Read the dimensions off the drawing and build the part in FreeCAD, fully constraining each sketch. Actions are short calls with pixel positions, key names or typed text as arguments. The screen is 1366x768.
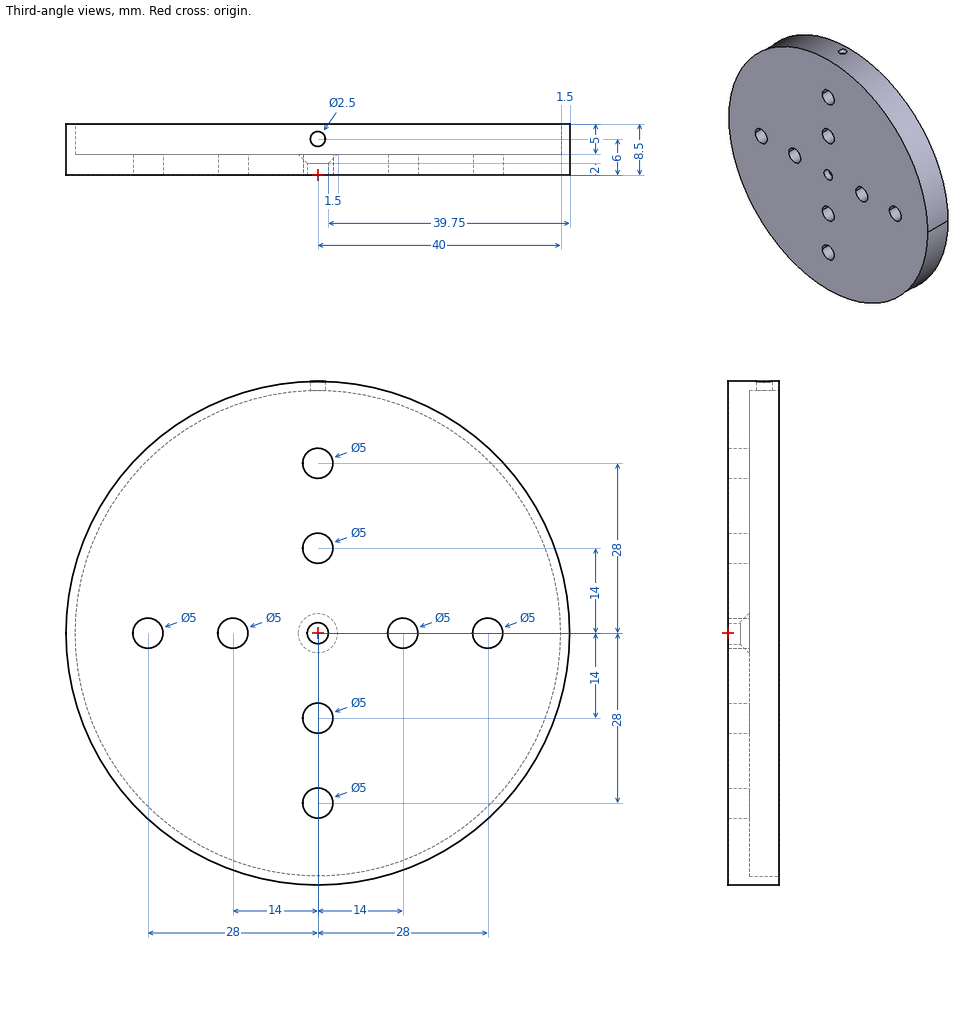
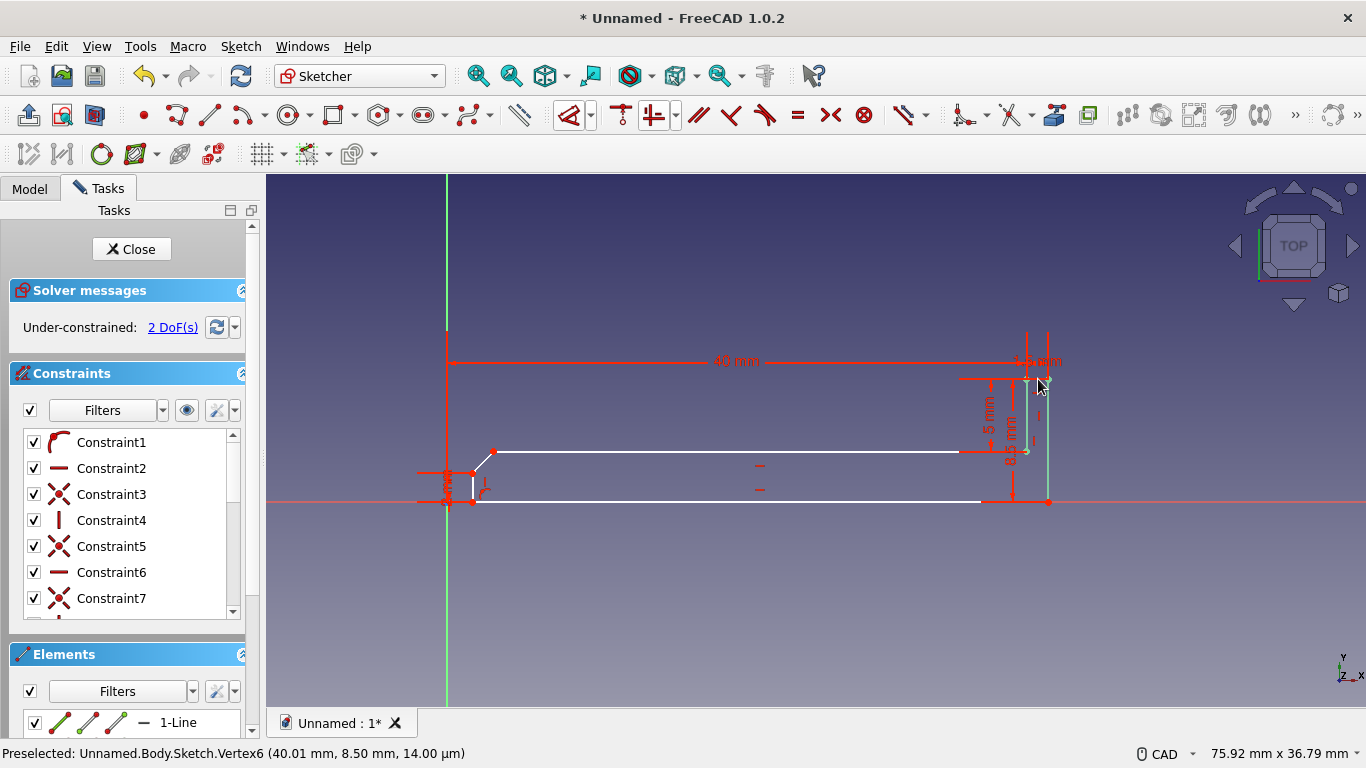
scroll(487, 458, up, 4)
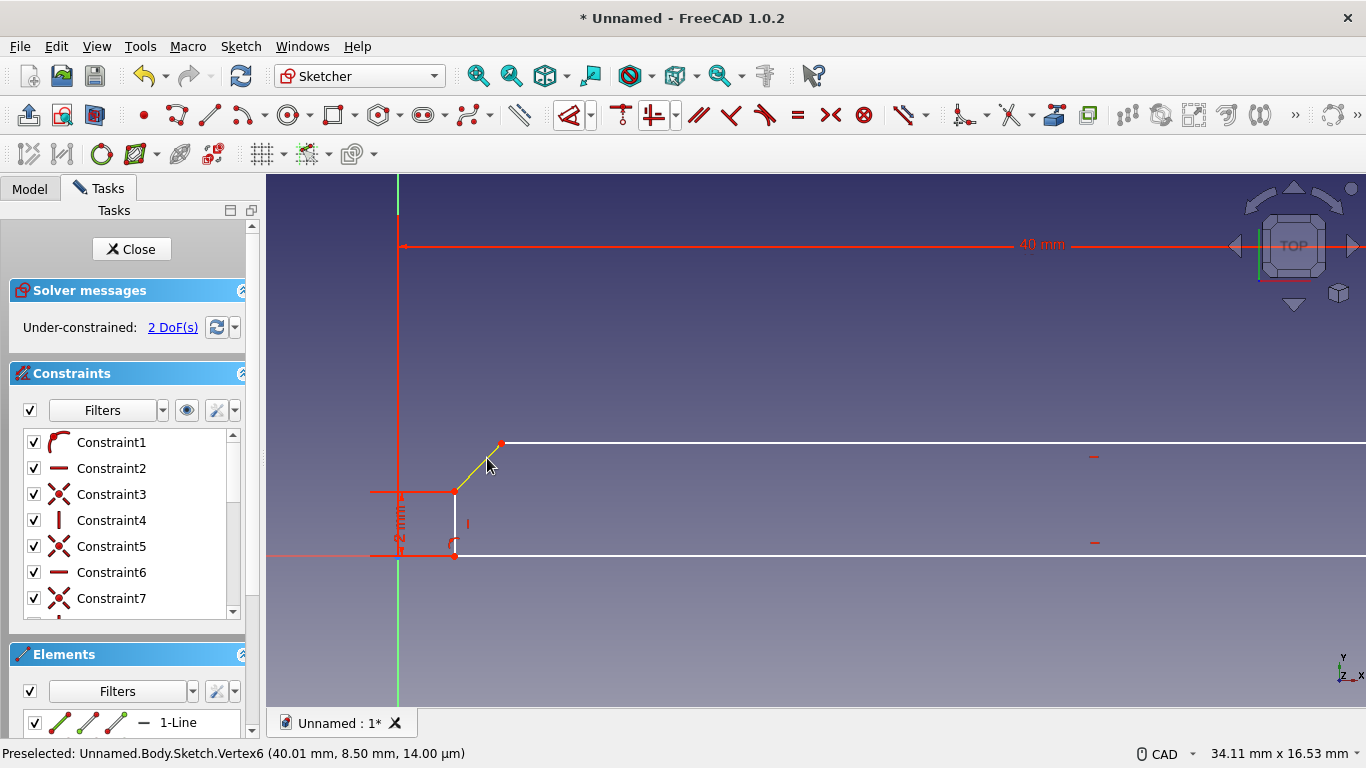
click(488, 458)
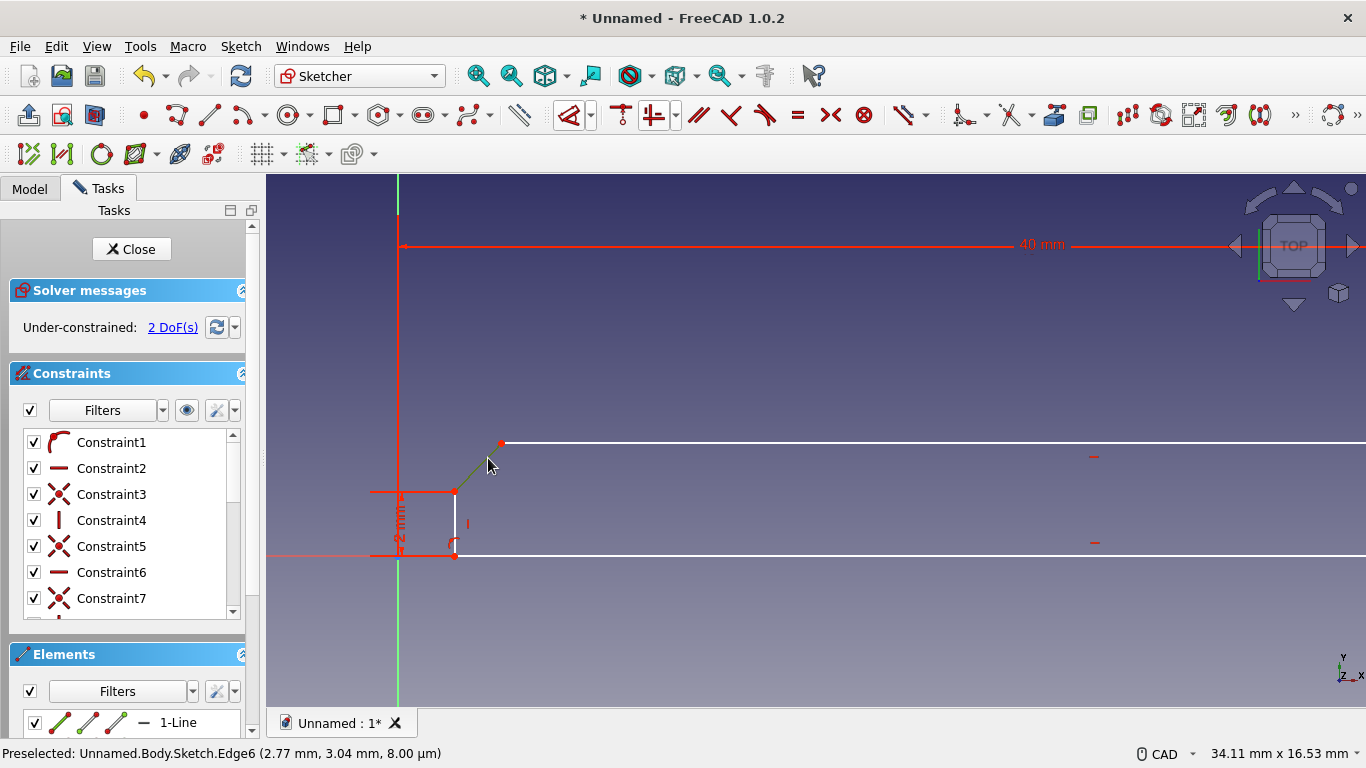
click(590, 116)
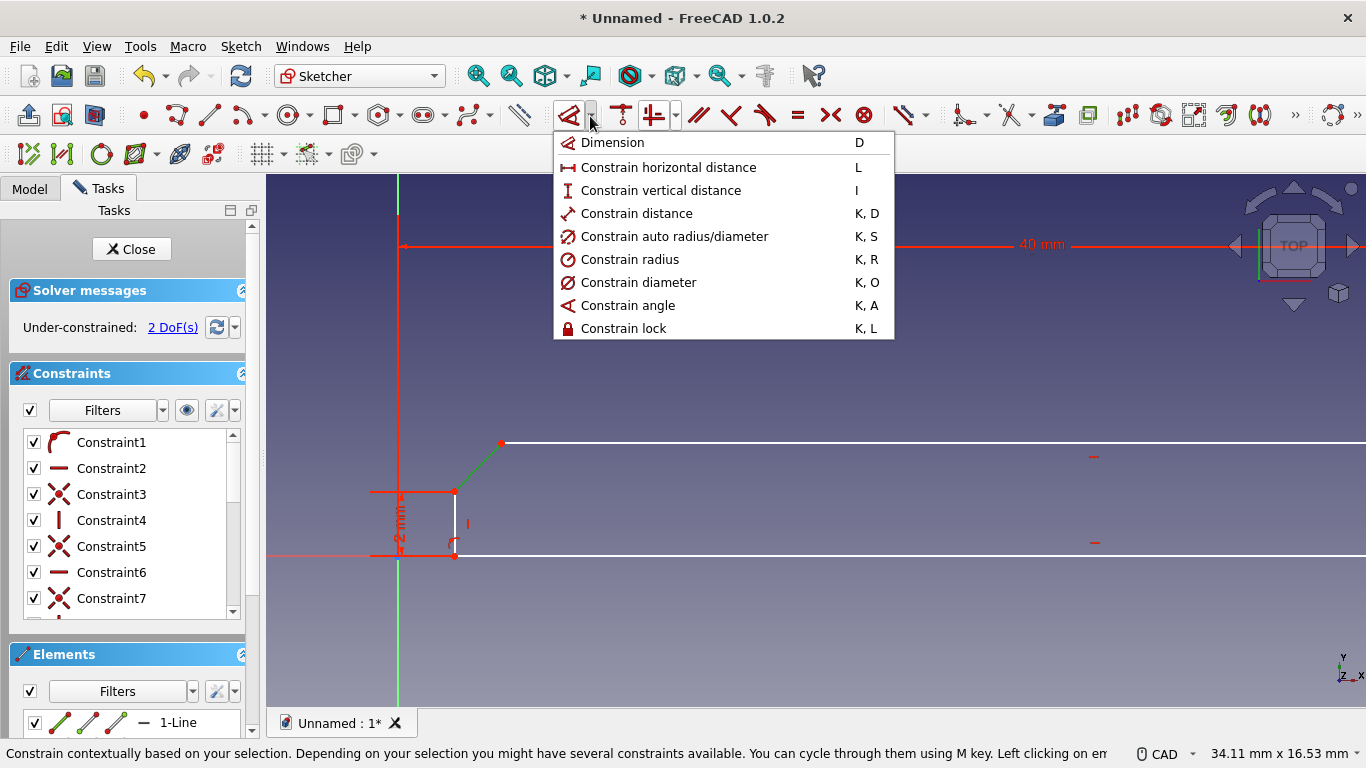
click(724, 168)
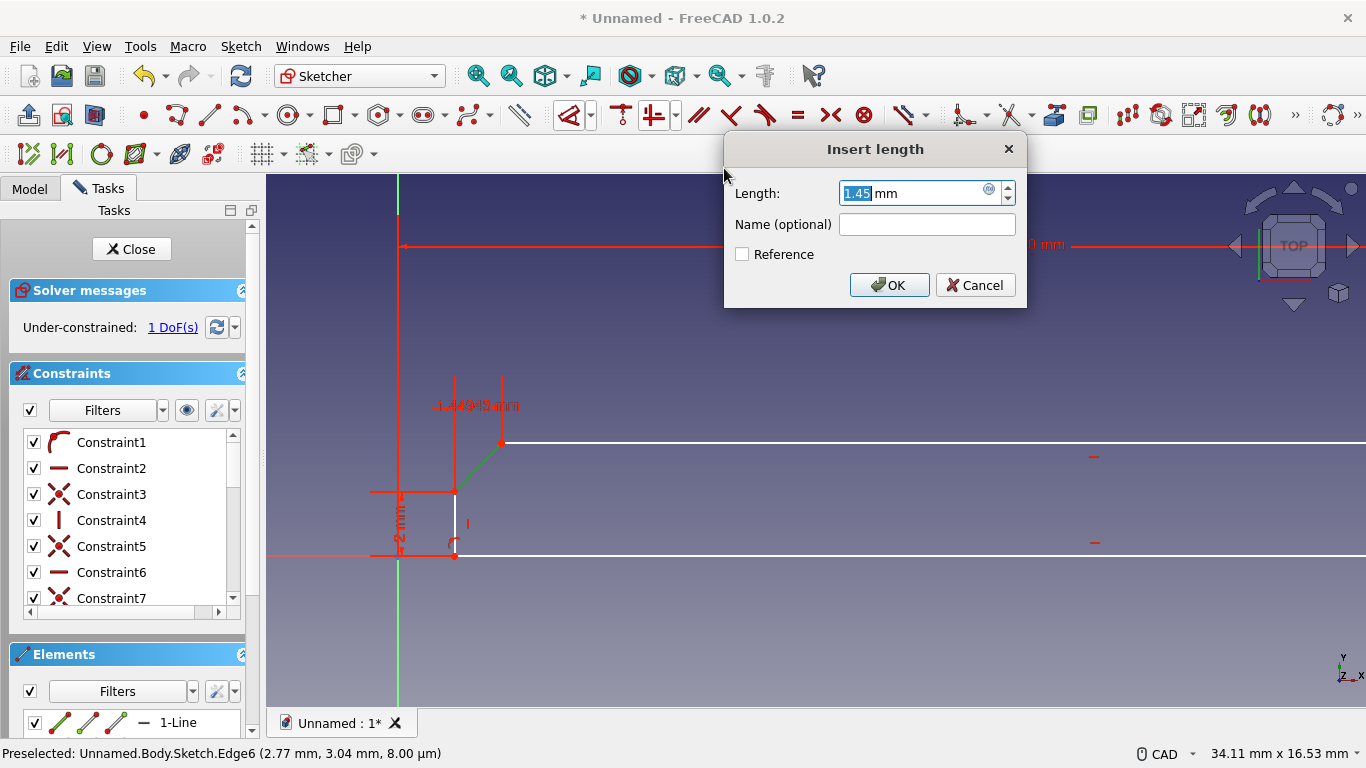
text(1.5)
key(Return)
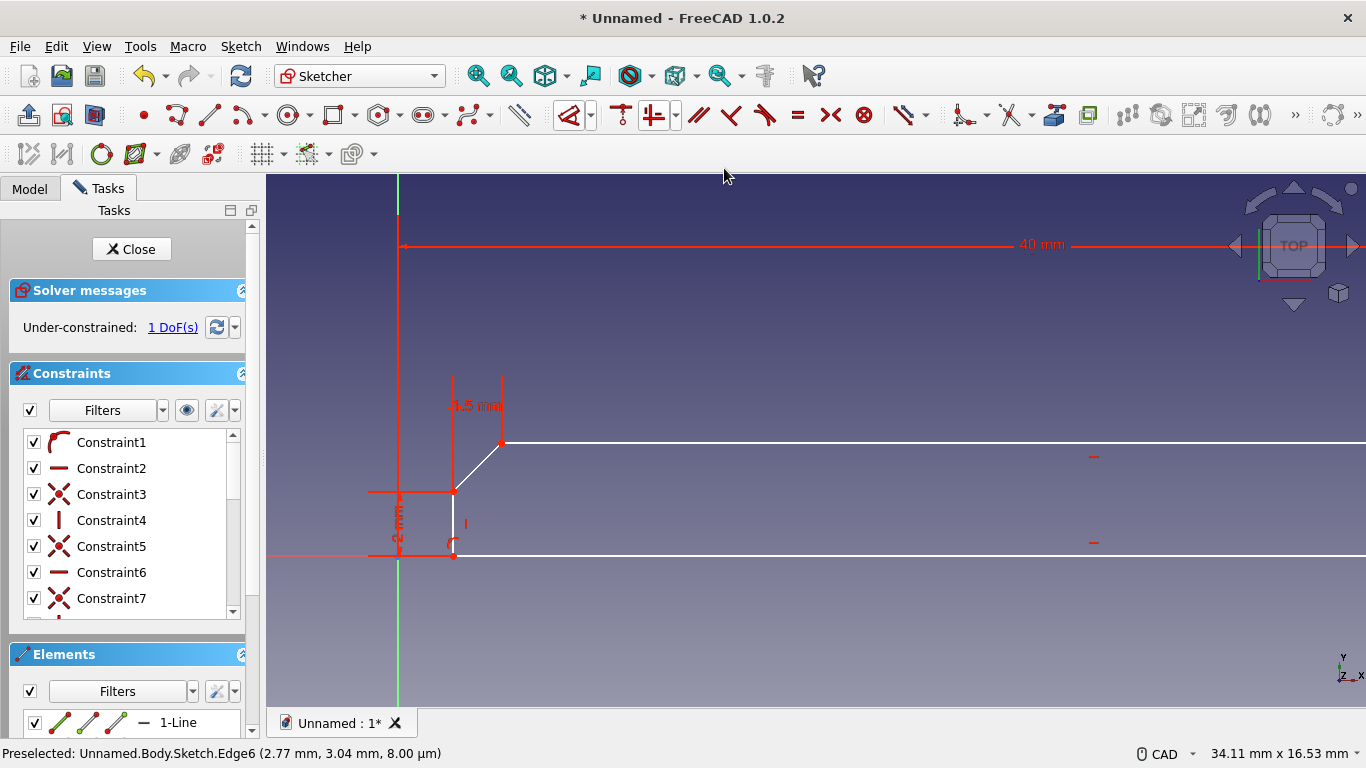
click(838, 556)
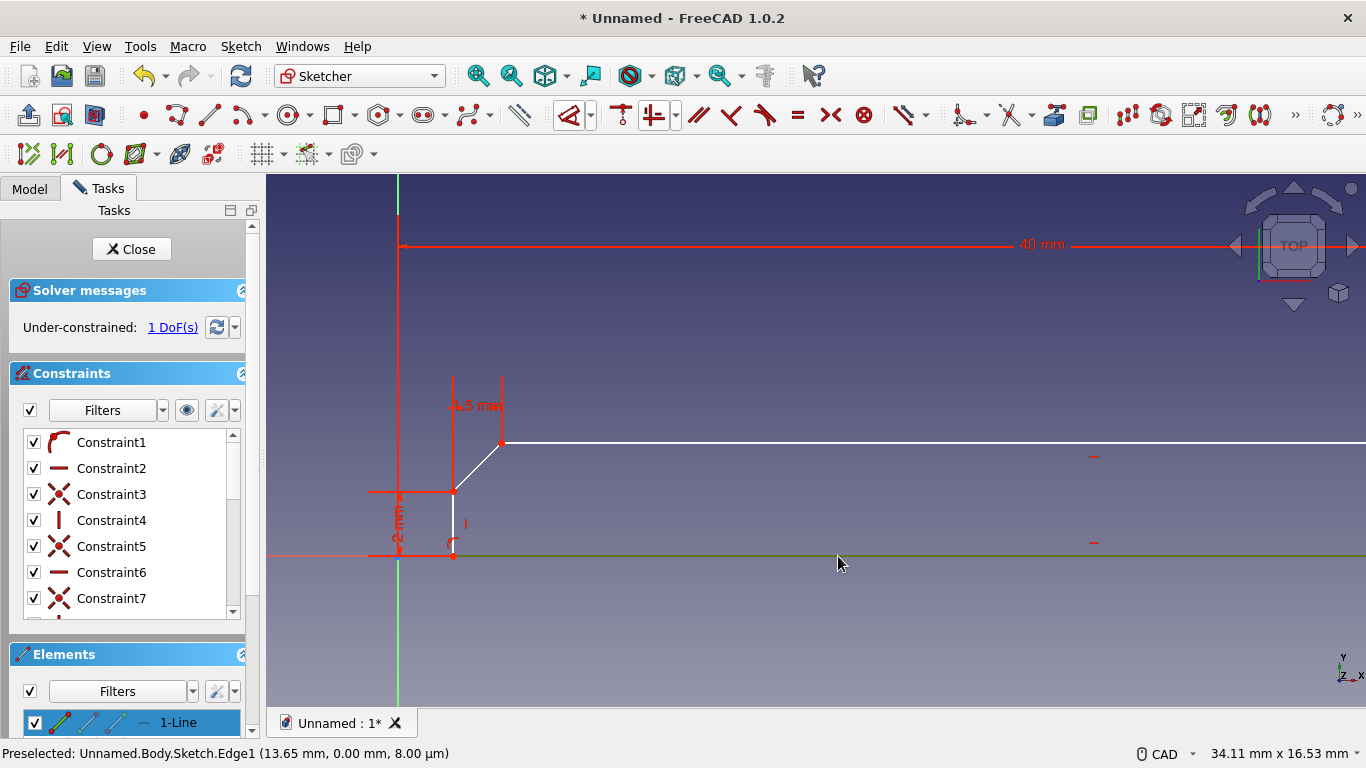
click(590, 116)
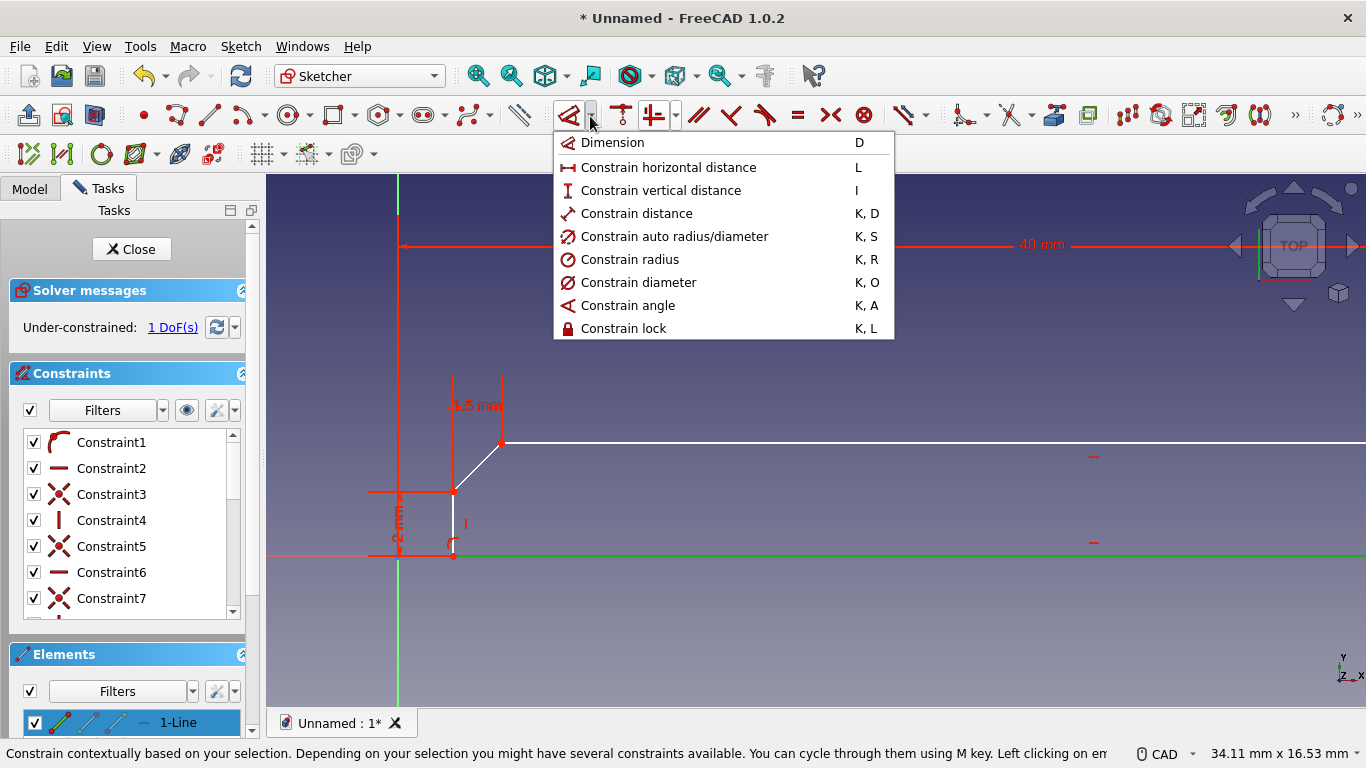
click(724, 168)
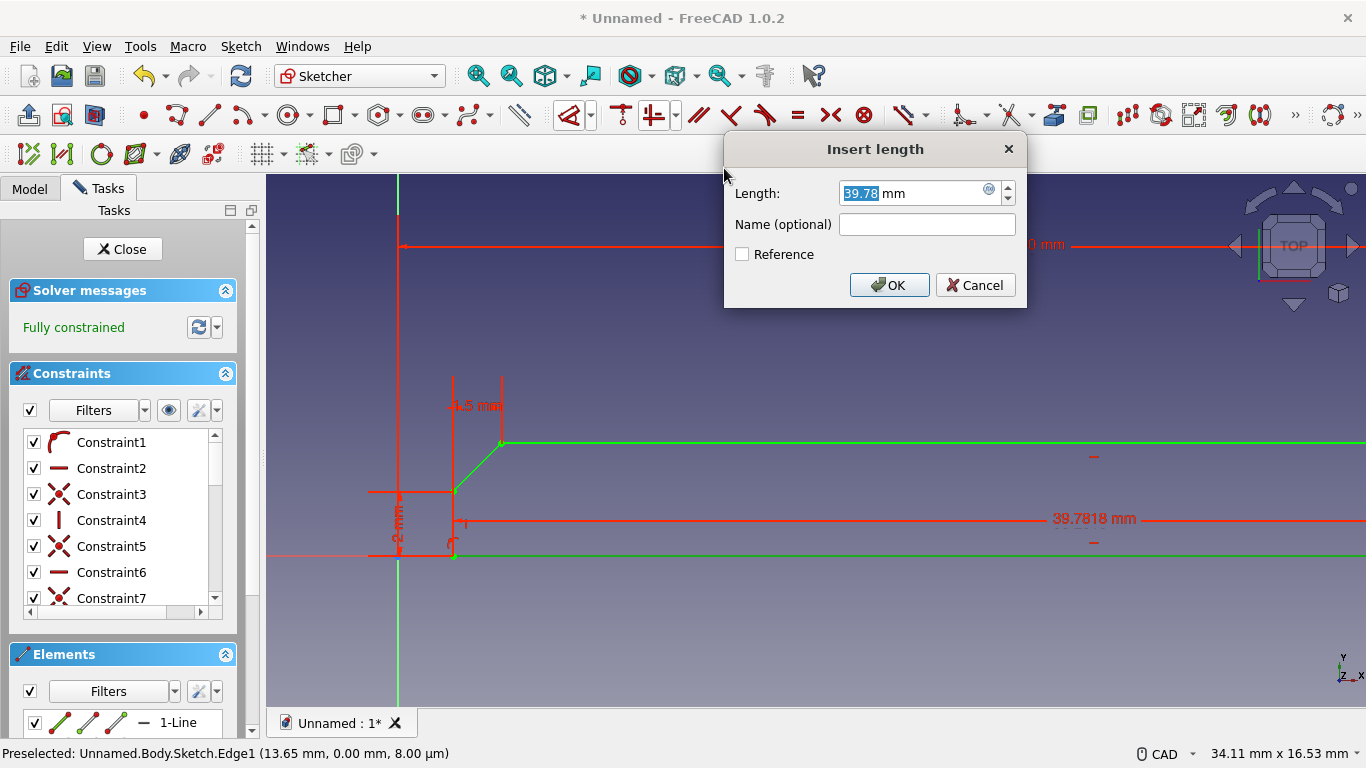
text(39.75)
key(Return)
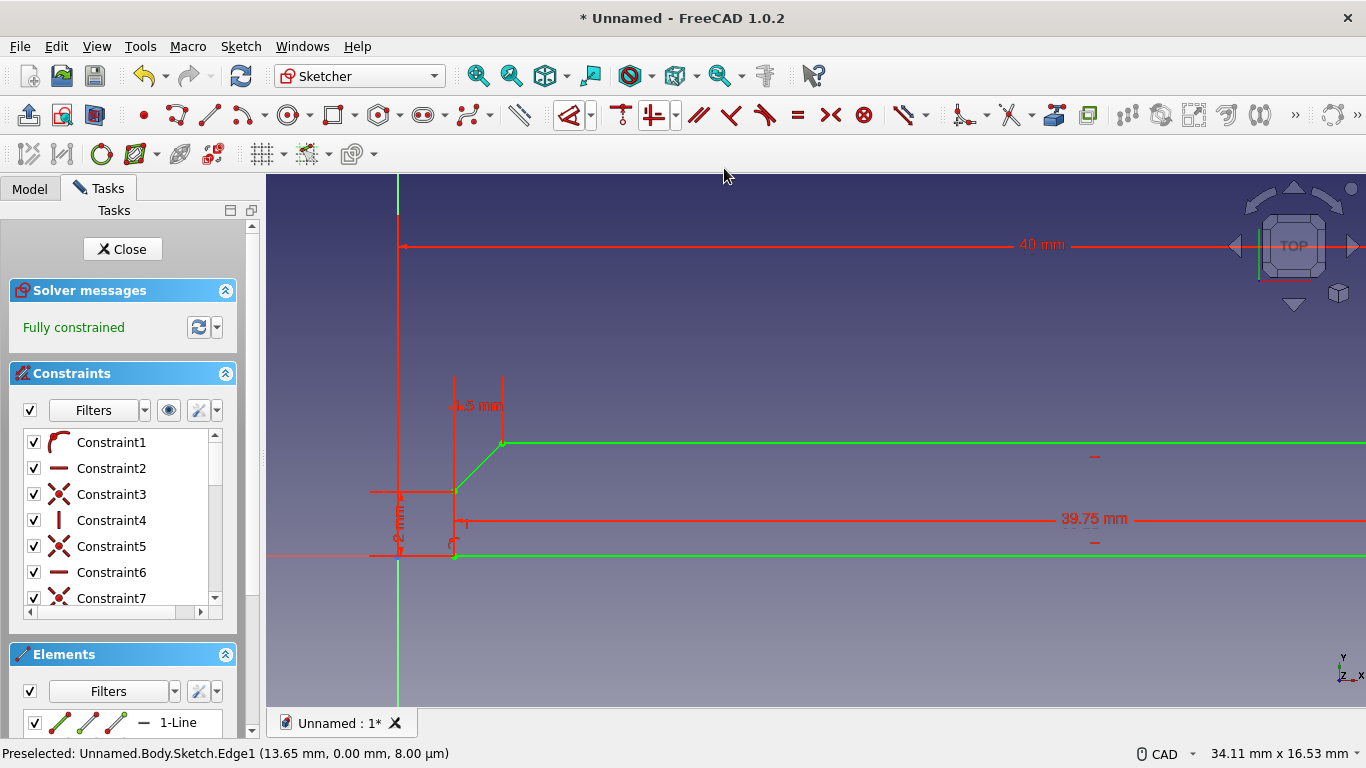
click(123, 249)